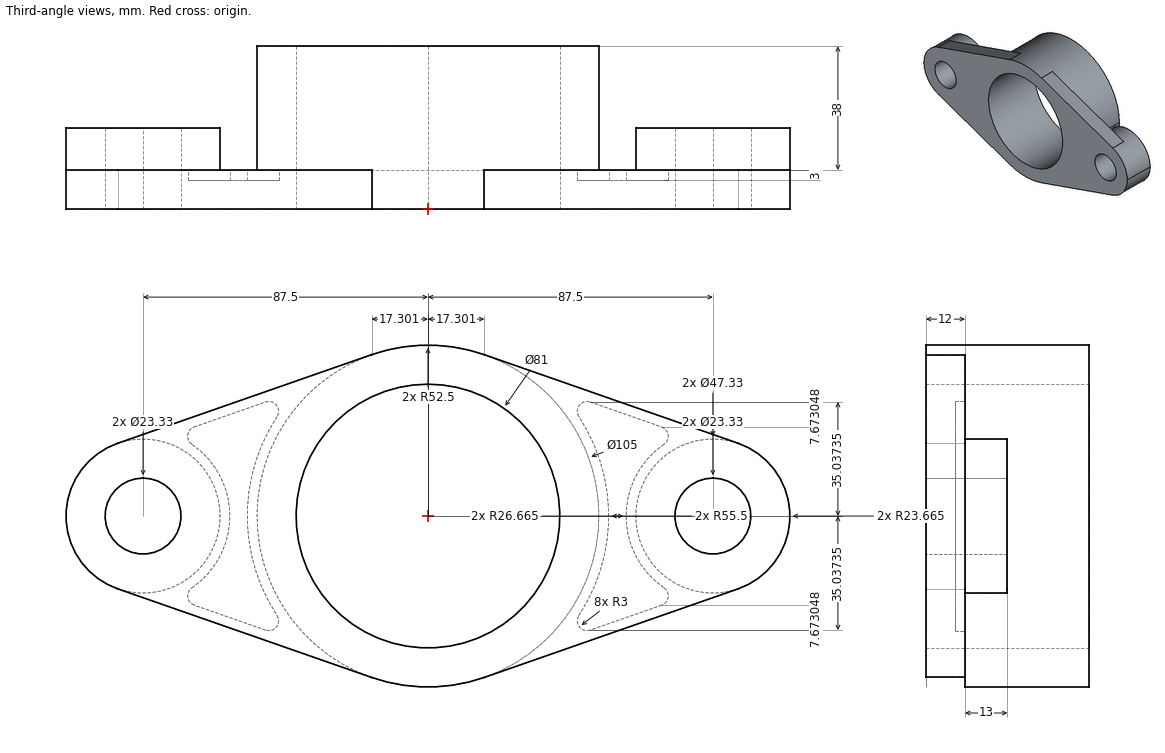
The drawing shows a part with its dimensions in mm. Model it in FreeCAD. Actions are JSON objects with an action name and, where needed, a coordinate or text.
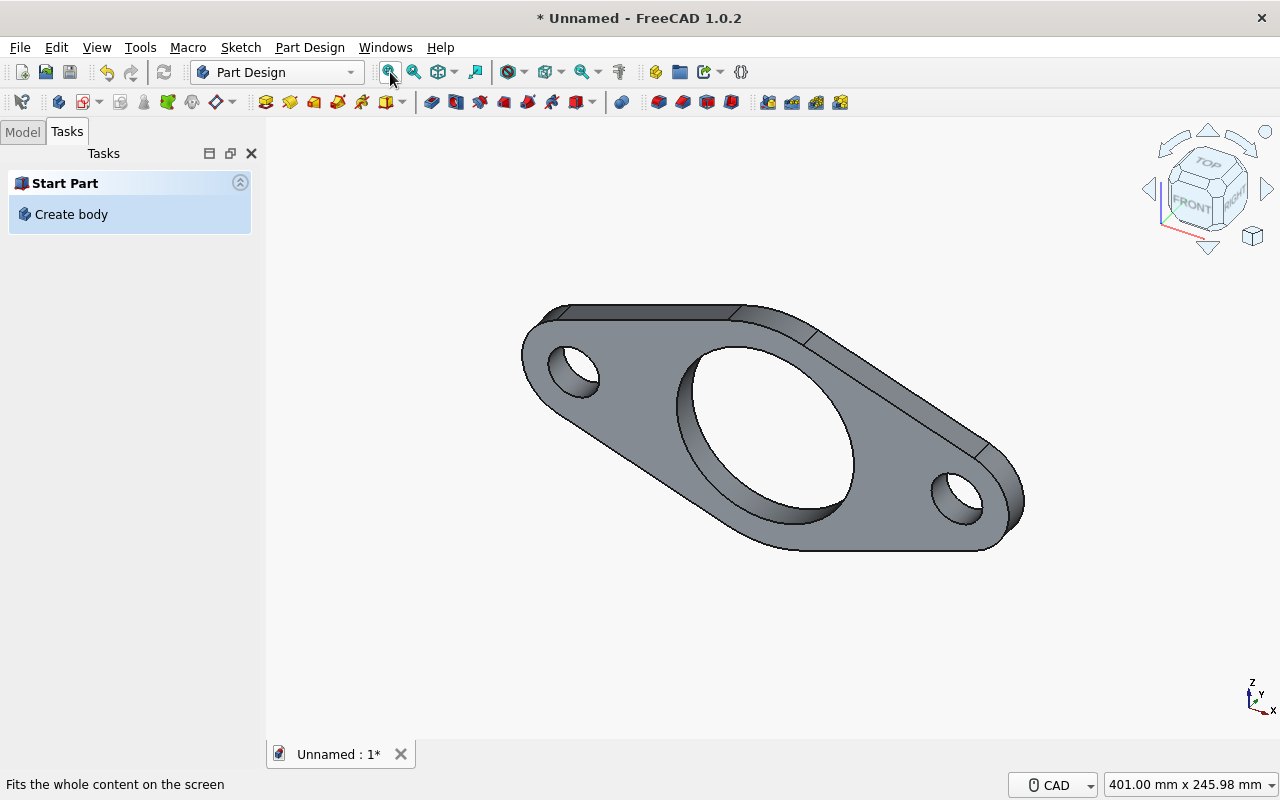
{"action": "key", "text": "4"}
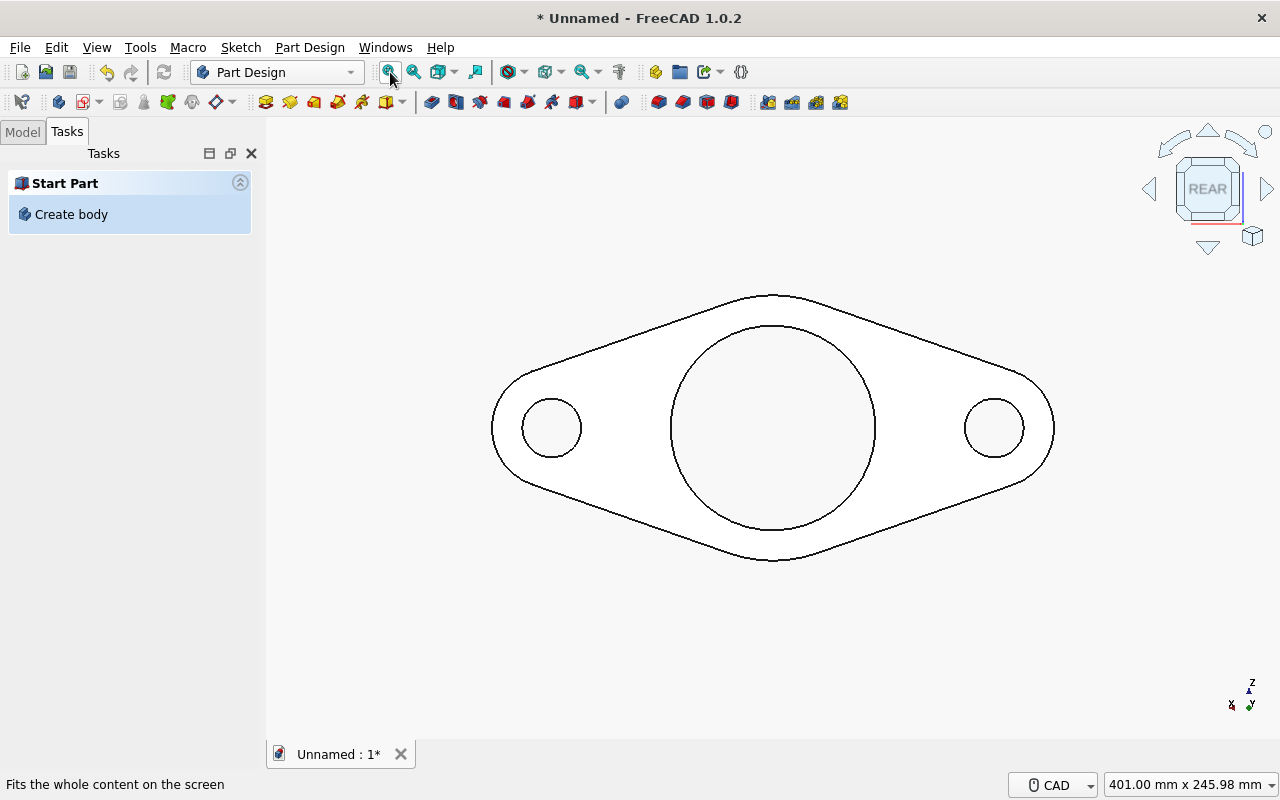
{"action": "left_click", "coordinate": [612, 389]}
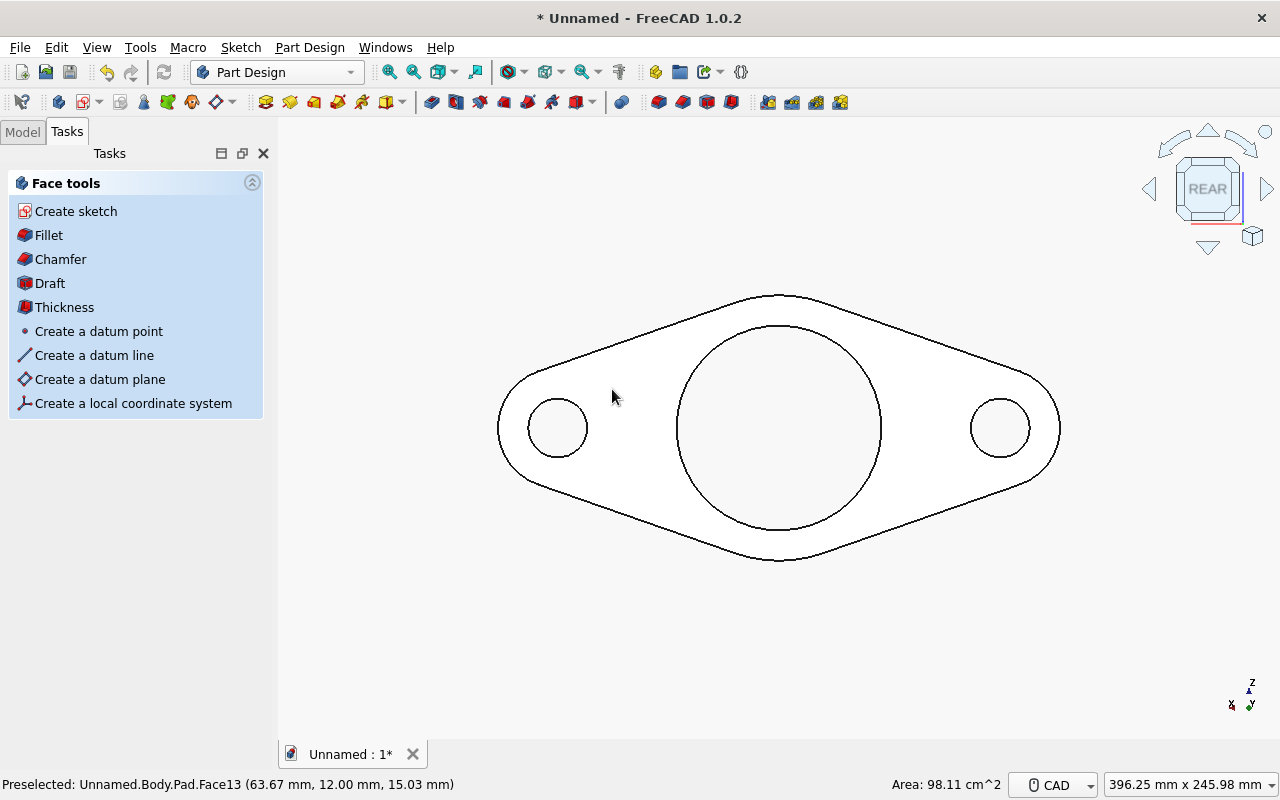
{"action": "left_click", "coordinate": [84, 102]}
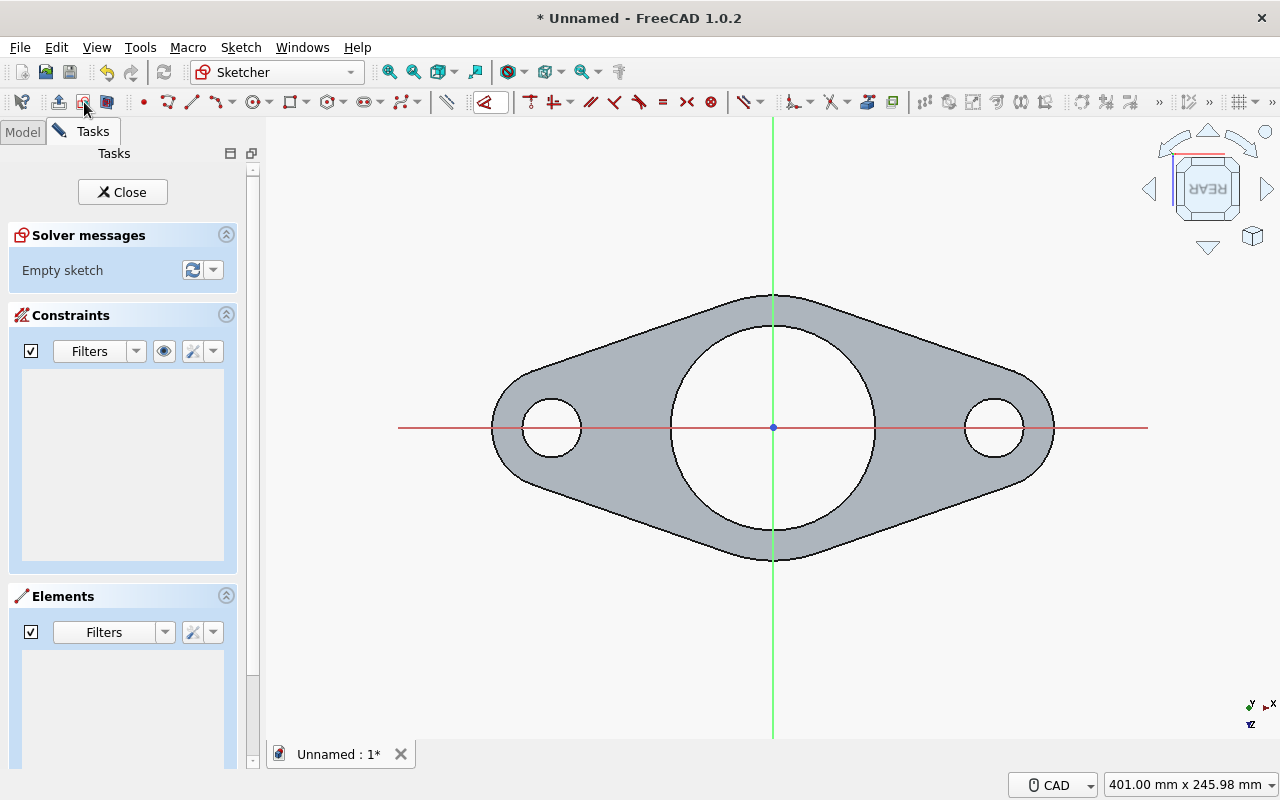
{"action": "scroll", "coordinate": [912, 428], "scroll_direction": "up", "scroll_amount": 2}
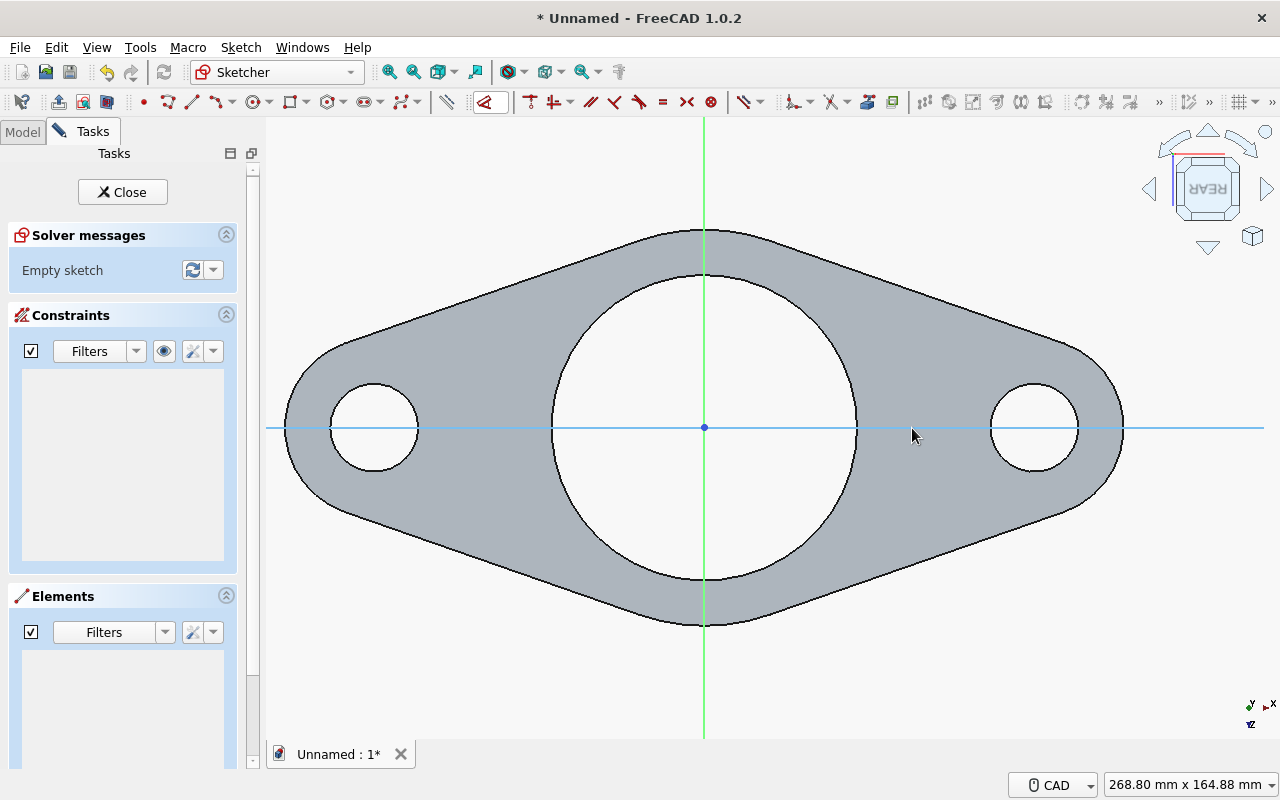
{"action": "left_click", "coordinate": [254, 102]}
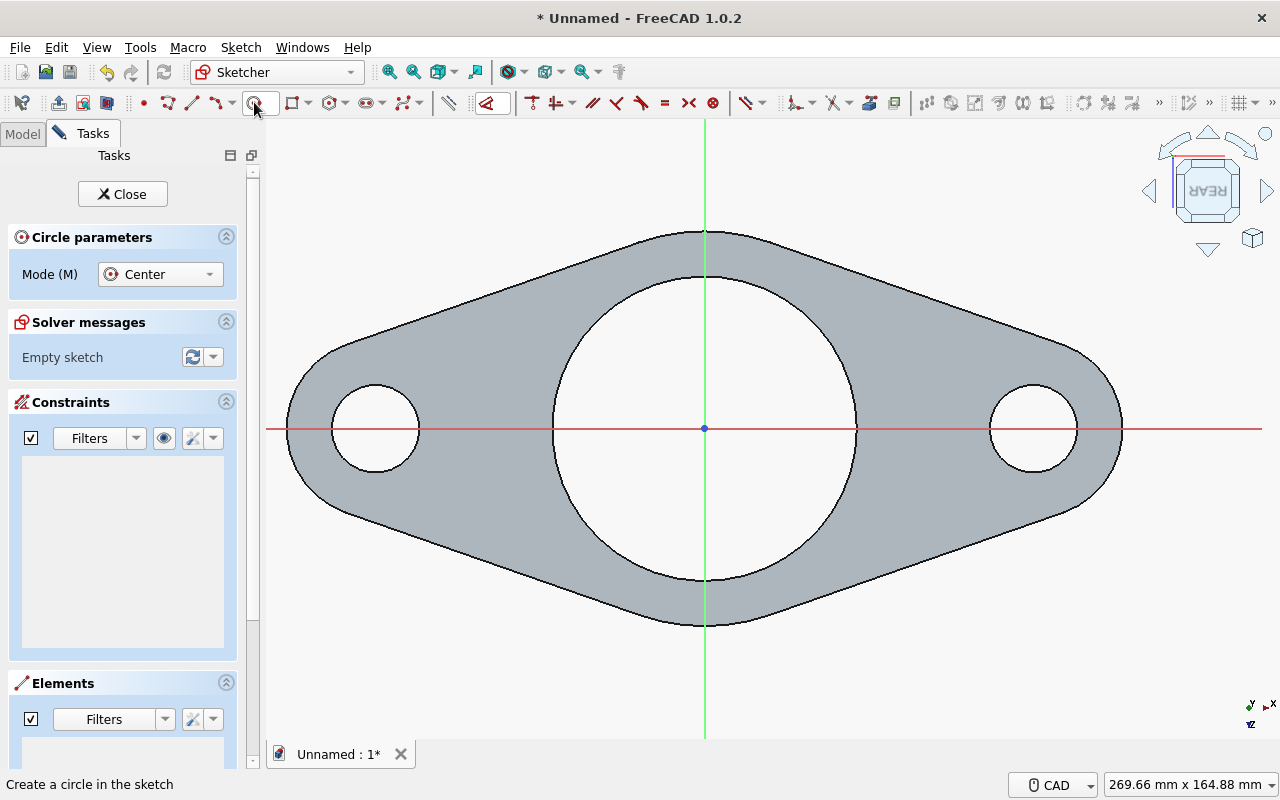
{"action": "left_click", "coordinate": [705, 429]}
{"action": "mouse_move", "coordinate": [844, 289]}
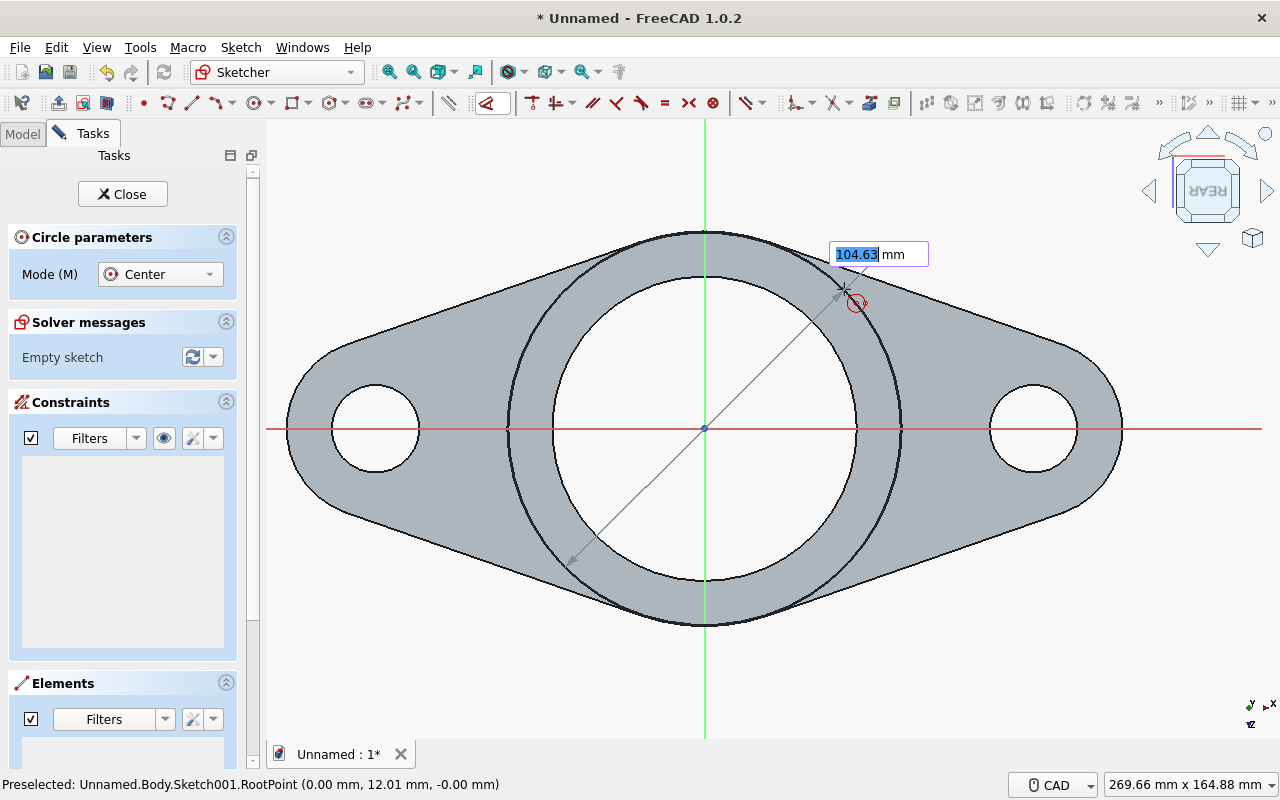
{"action": "type", "text": "105"}
{"action": "key", "text": "Return"}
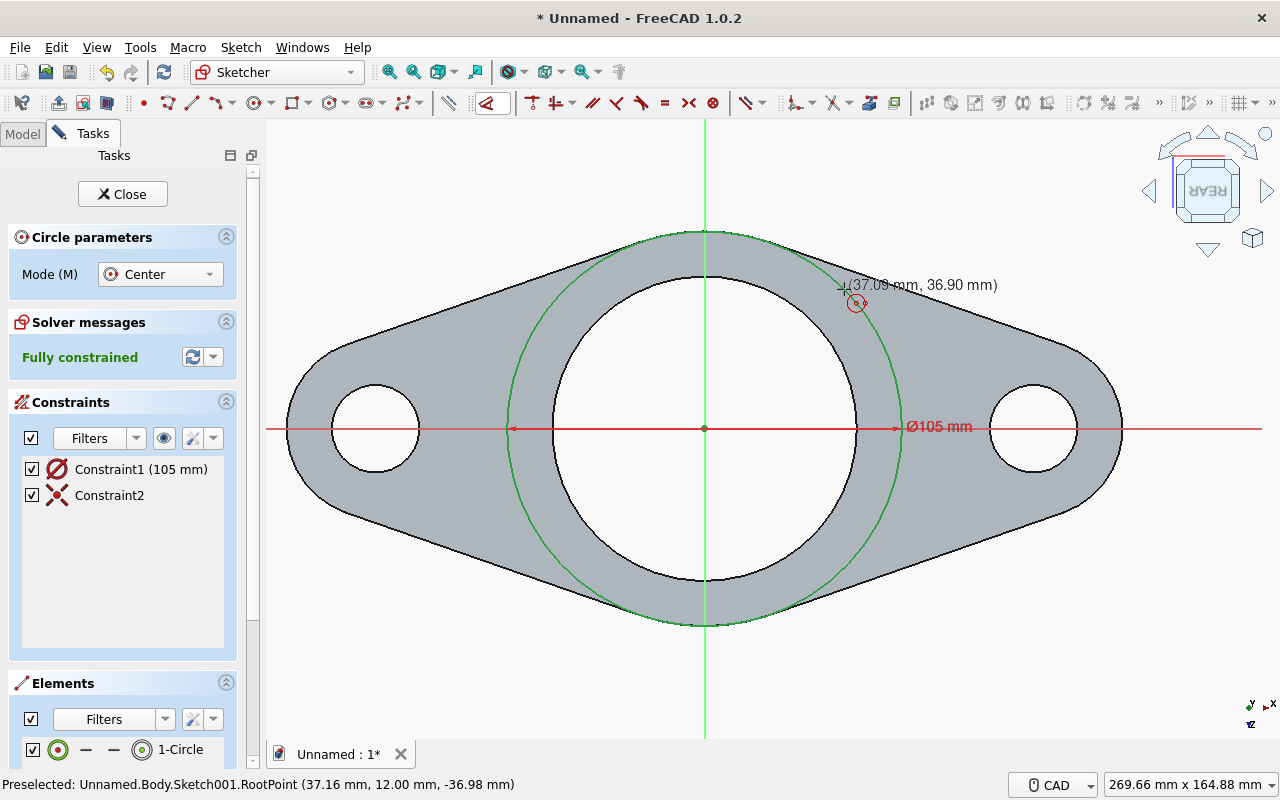
{"action": "left_click", "coordinate": [705, 429]}
{"action": "mouse_move", "coordinate": [812, 321]}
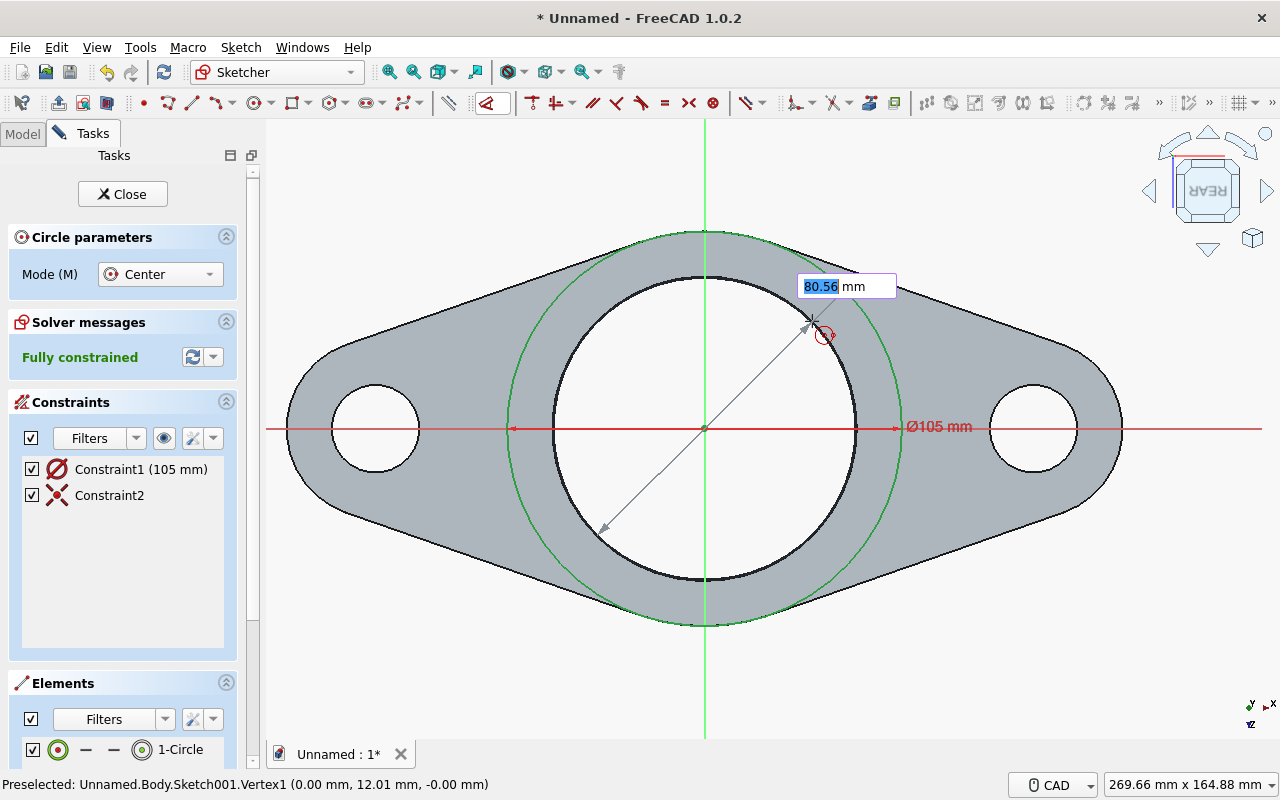
{"action": "type", "text": "81"}
{"action": "key", "text": "Return"}
{"action": "key", "text": "Escape"}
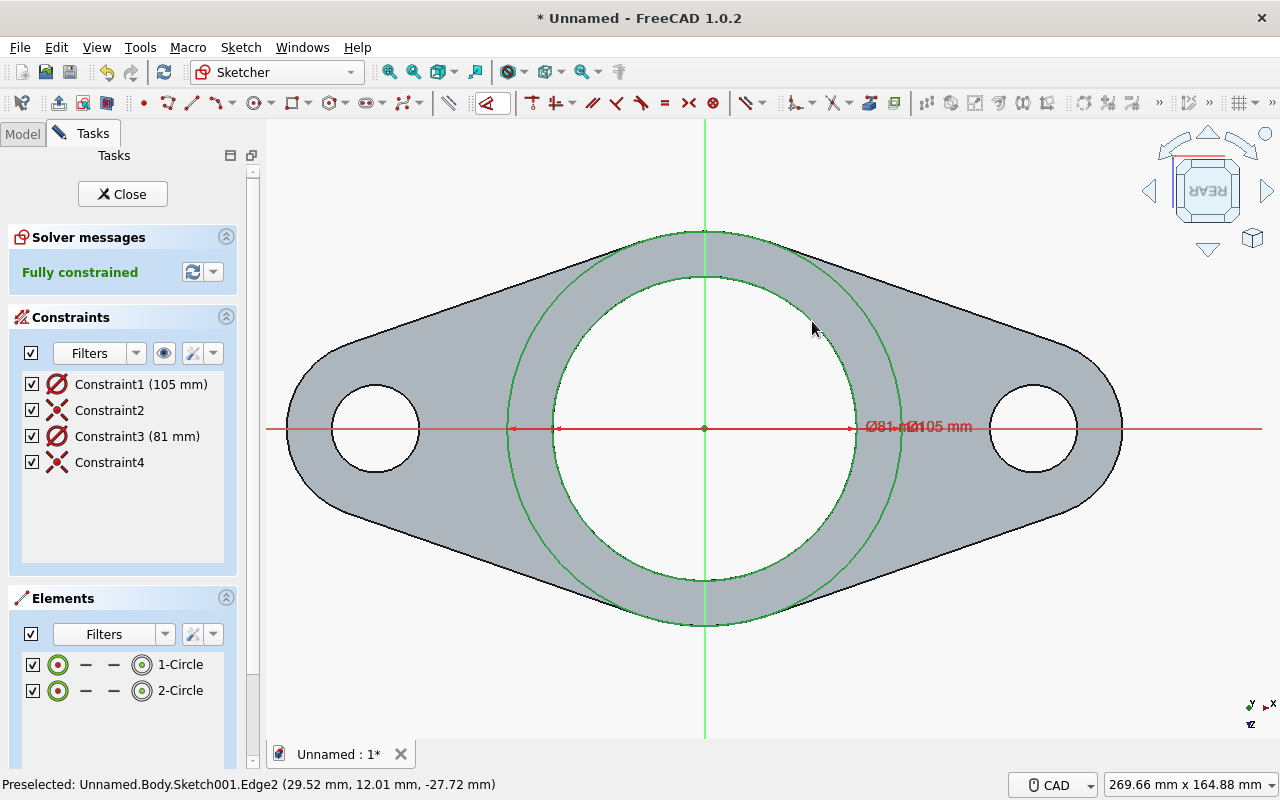
{"action": "left_click", "coordinate": [123, 194]}